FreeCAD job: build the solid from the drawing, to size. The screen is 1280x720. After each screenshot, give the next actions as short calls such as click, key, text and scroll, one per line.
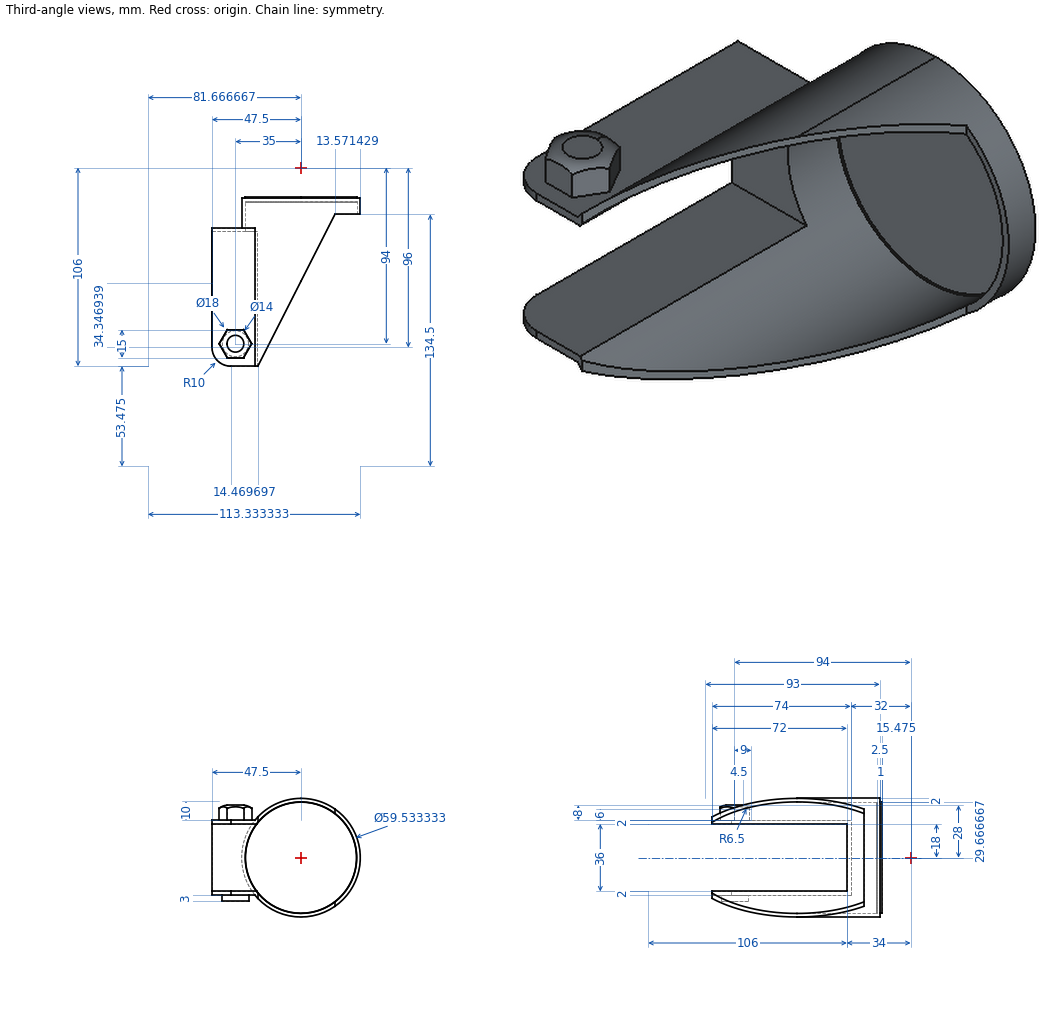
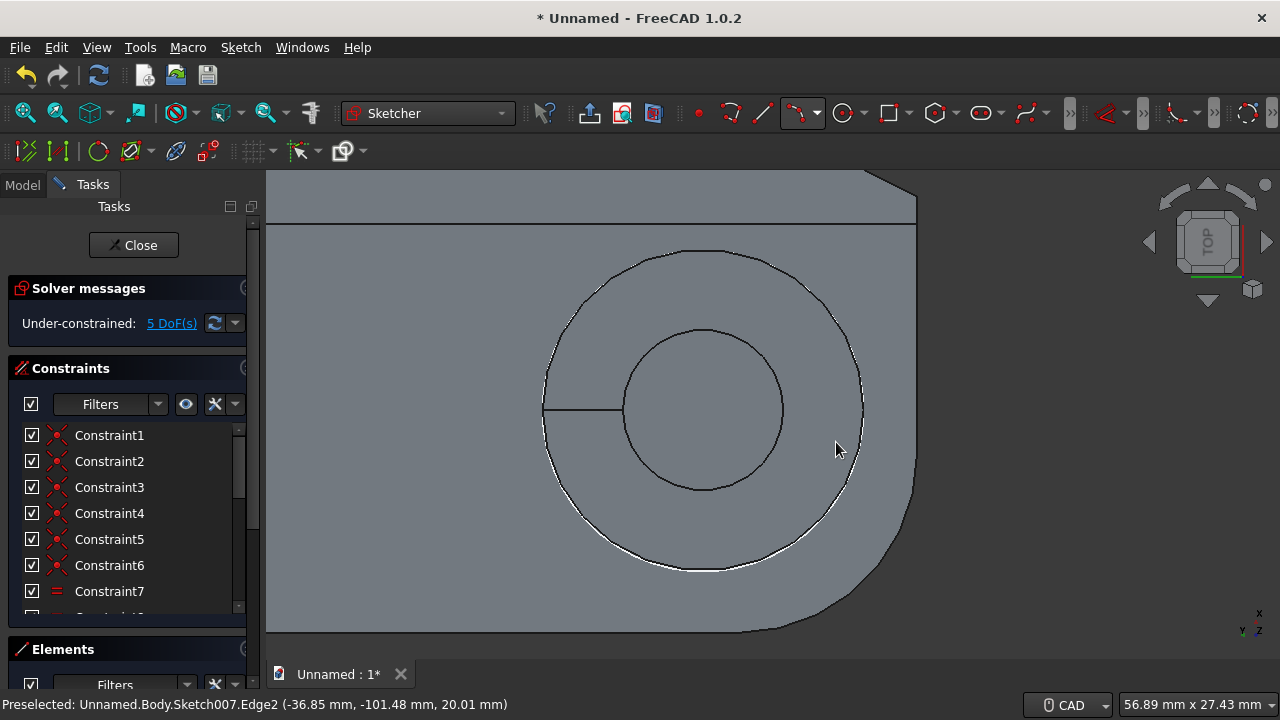
key(v)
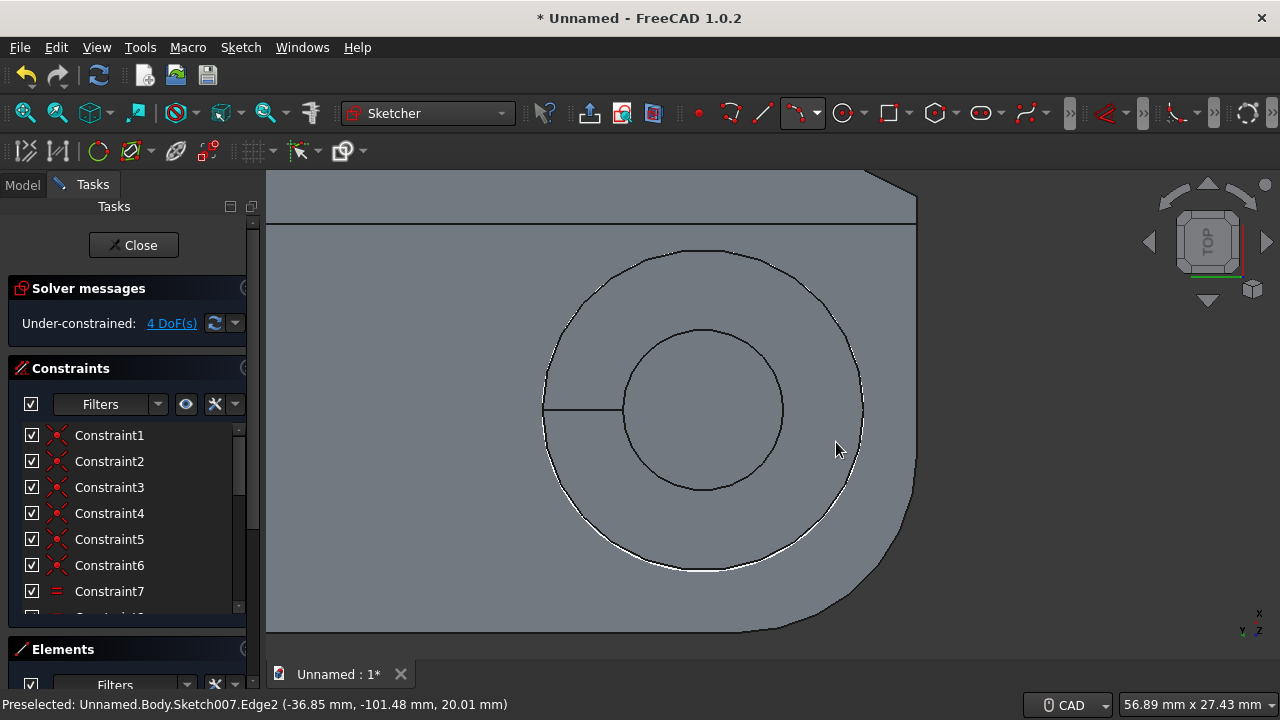
key(d)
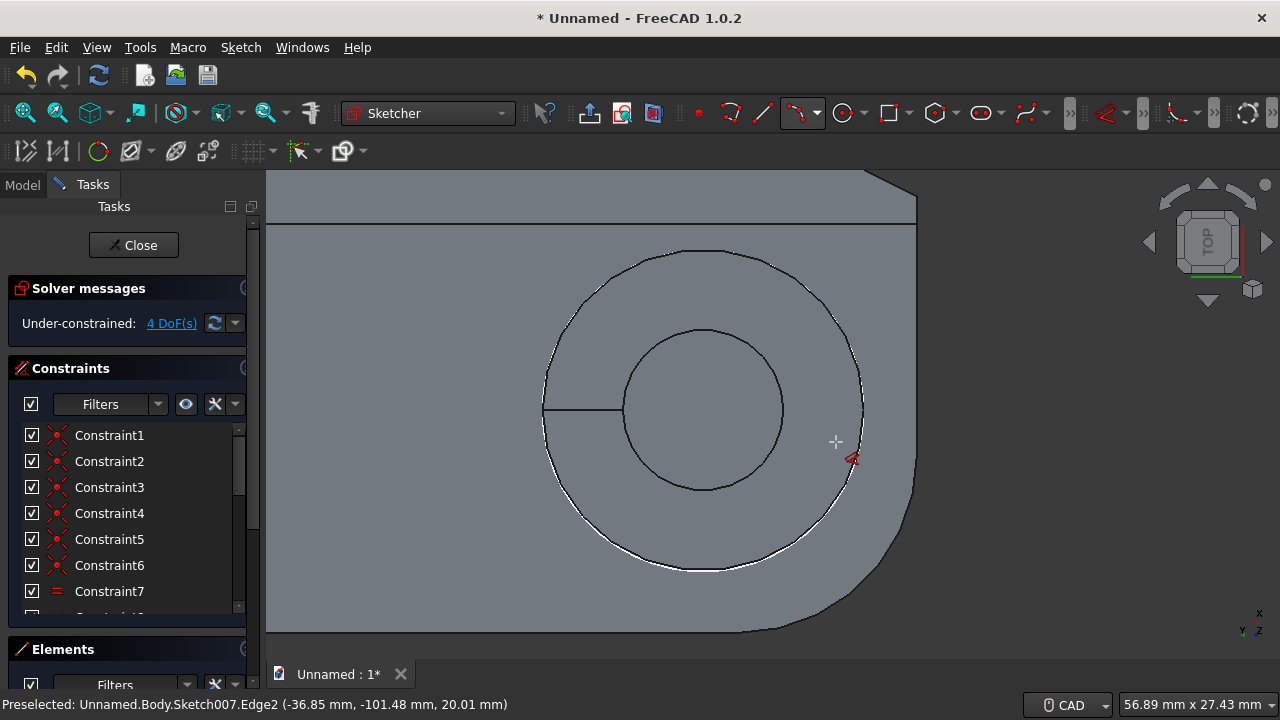
scroll(816, 297, up, 4)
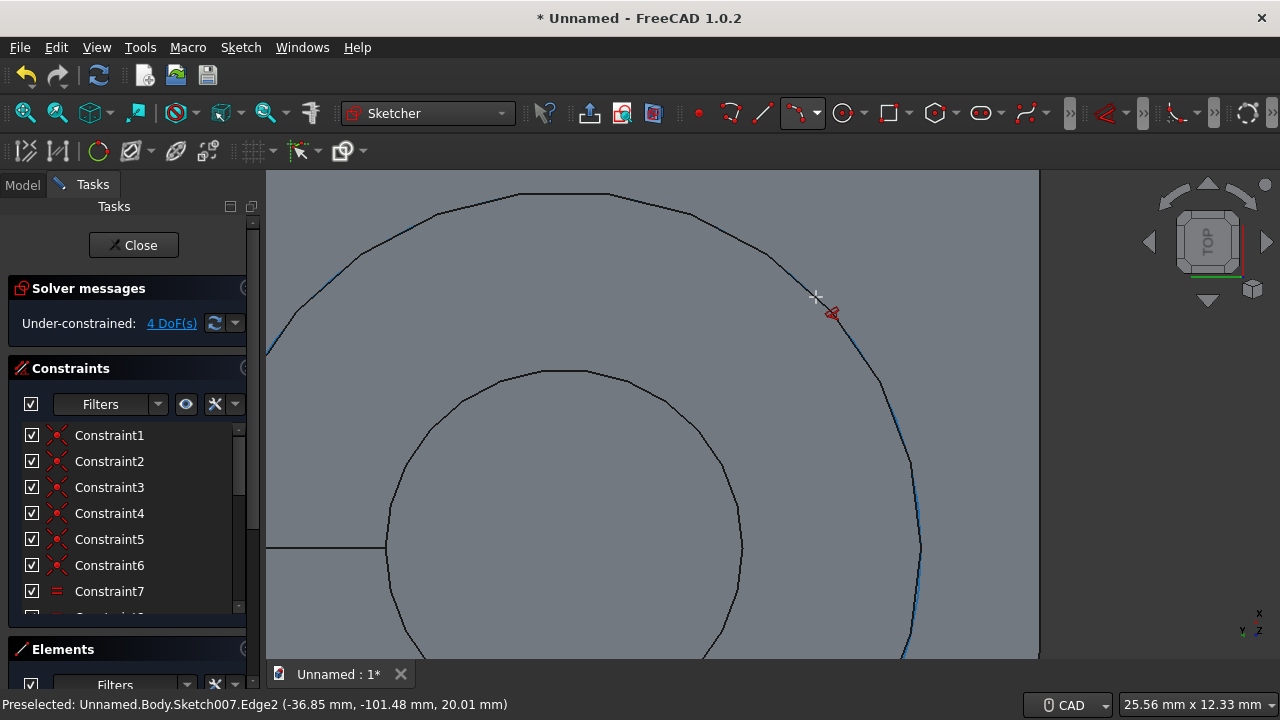
click(816, 297)
click(839, 274)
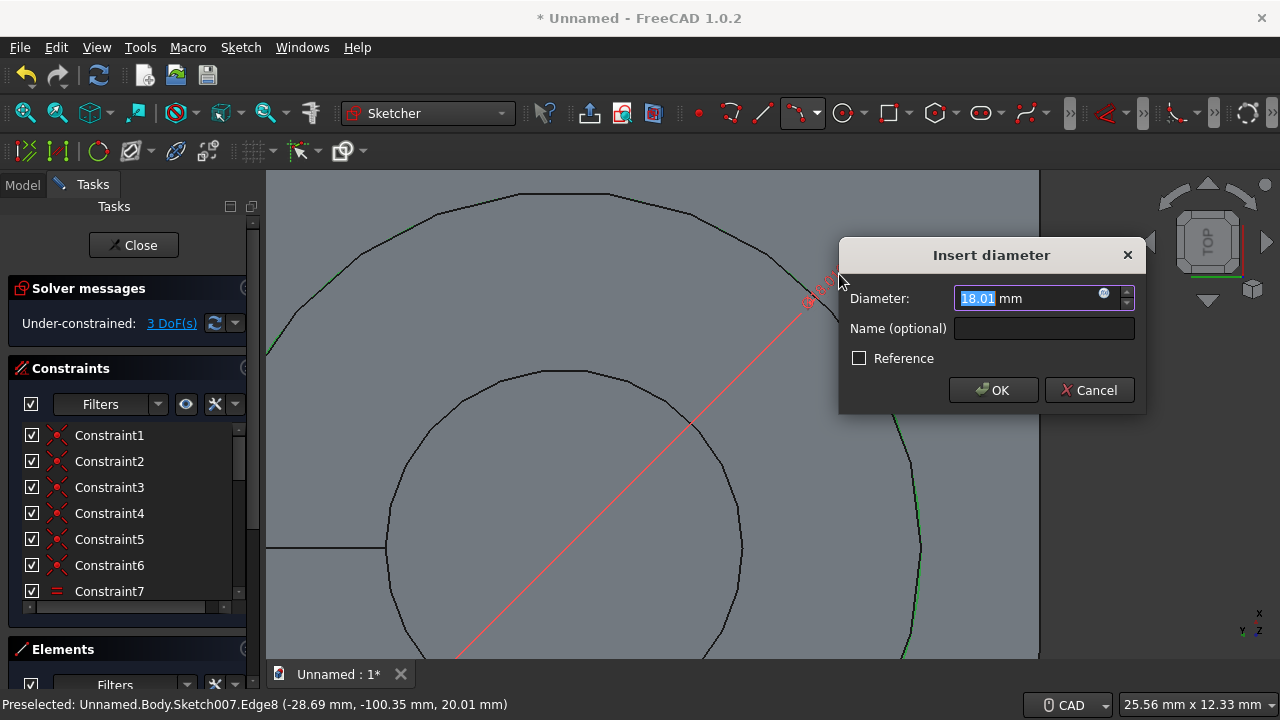
text(18)
key(Return)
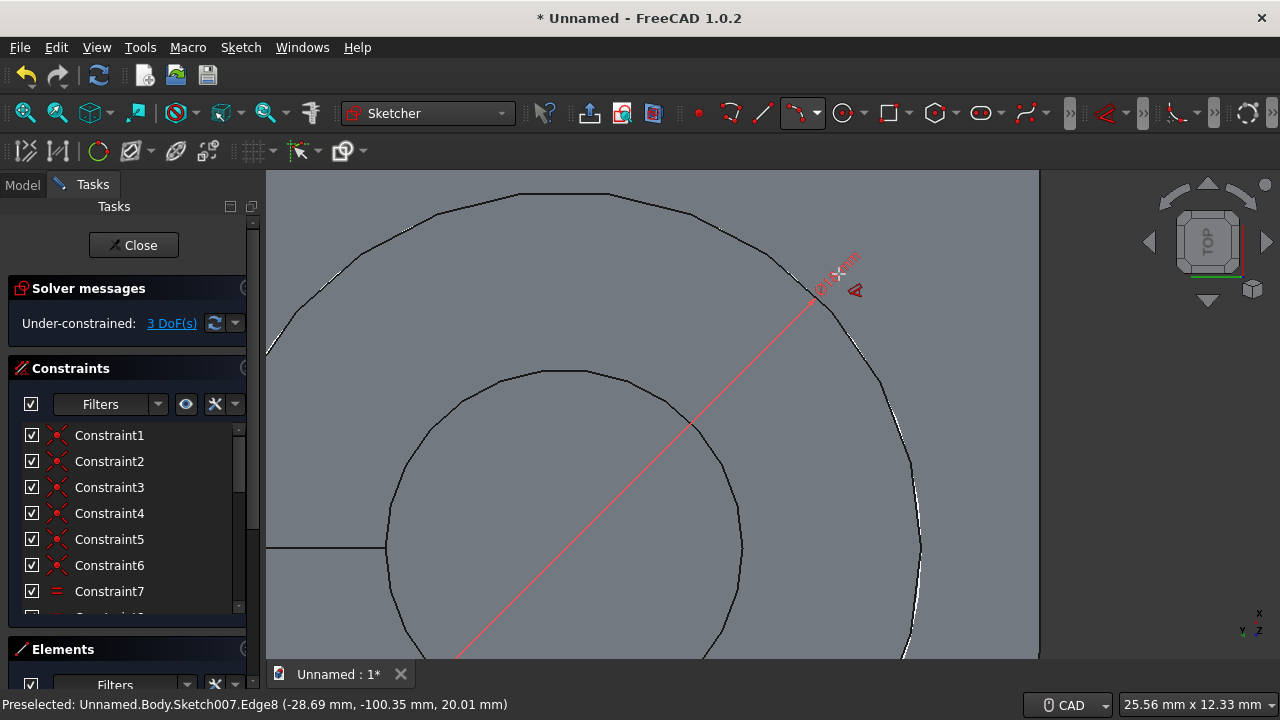
scroll(819, 305, down, 4)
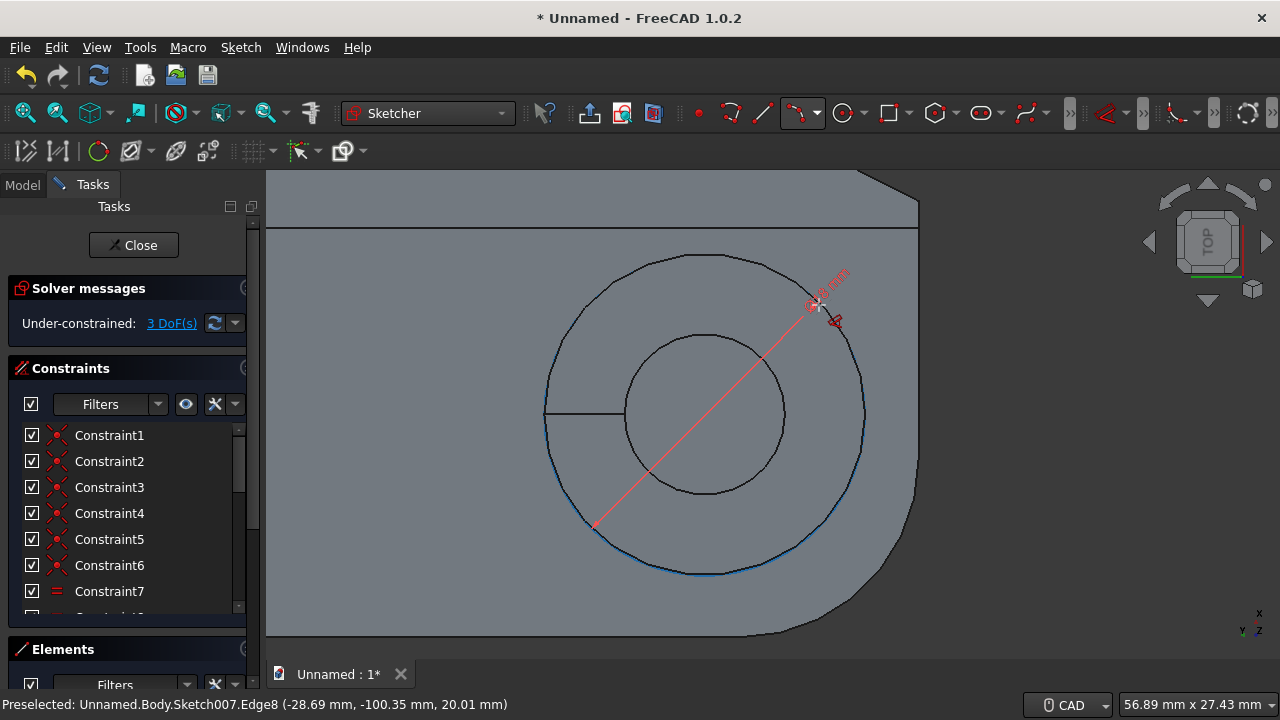
click(571, 338)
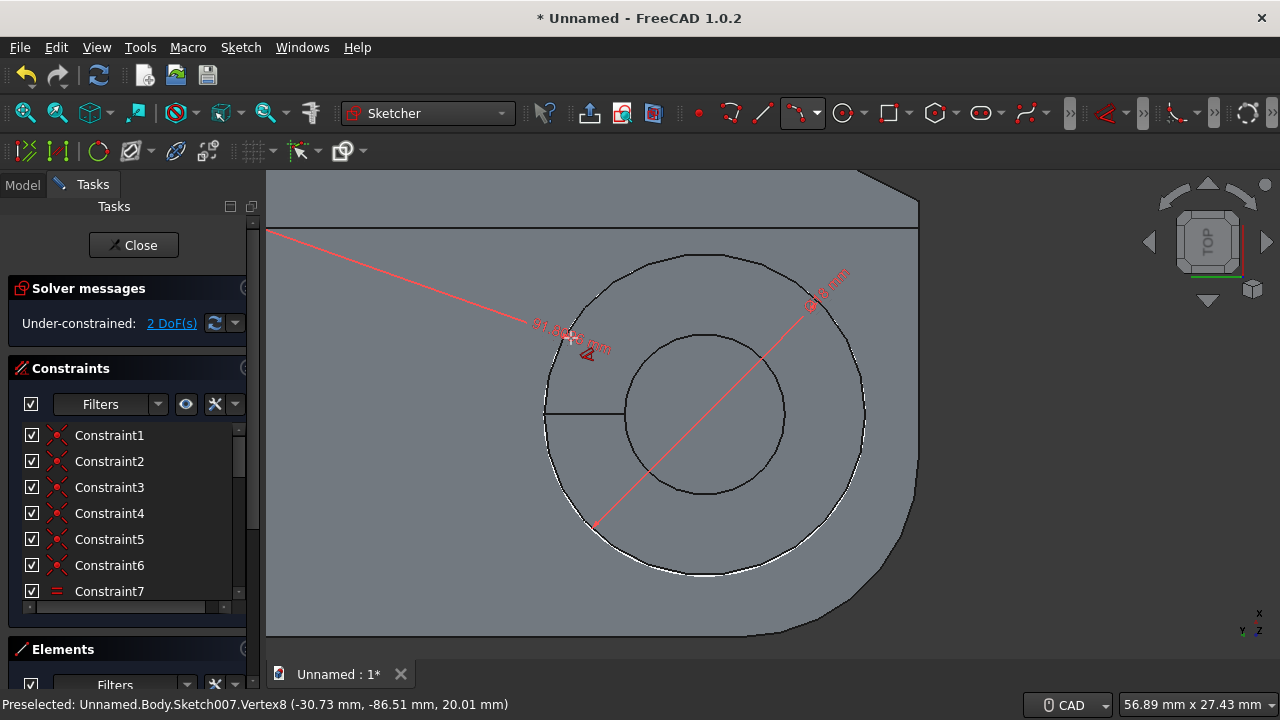
click(838, 492)
click(705, 526)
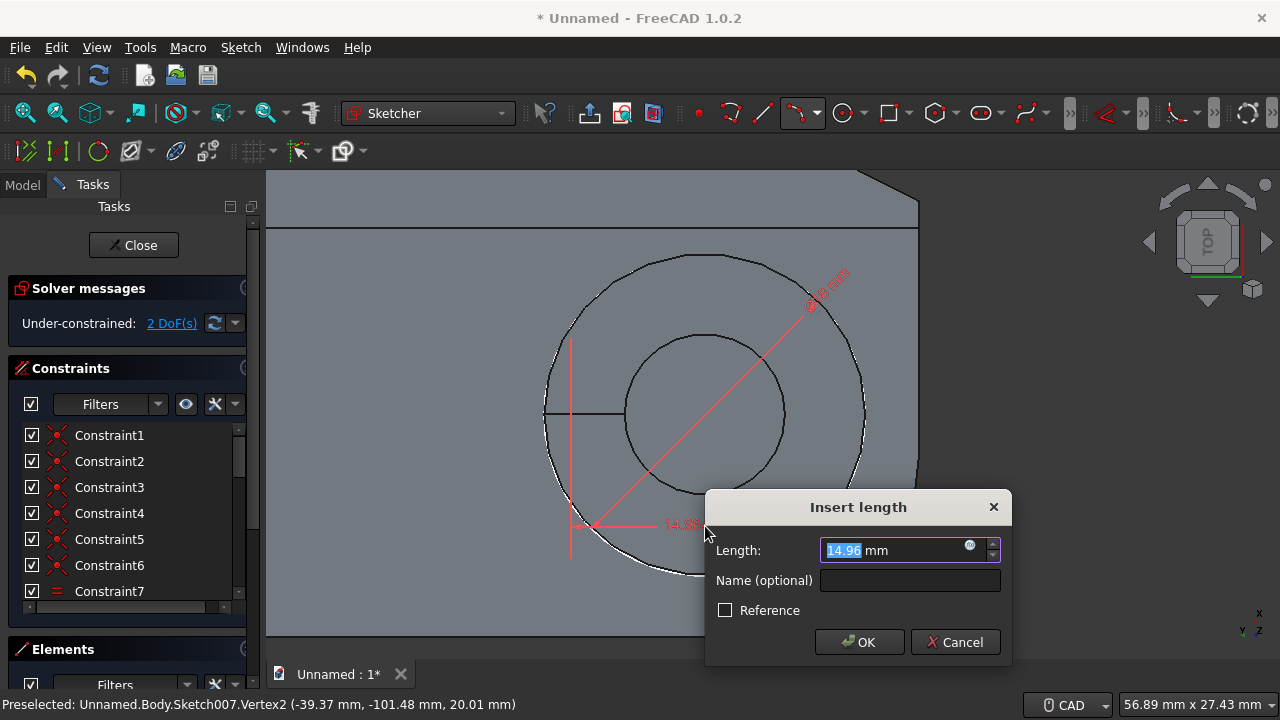
text(15)
key(Return)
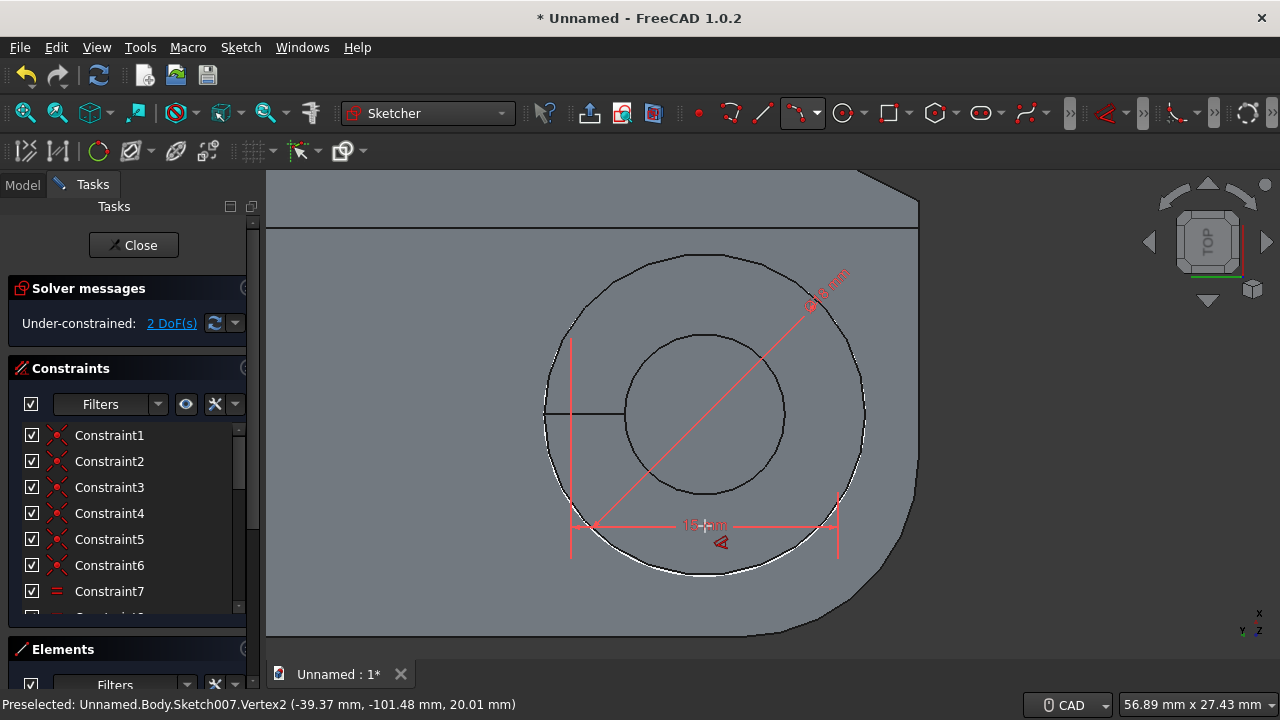
click(705, 416)
click(499, 450)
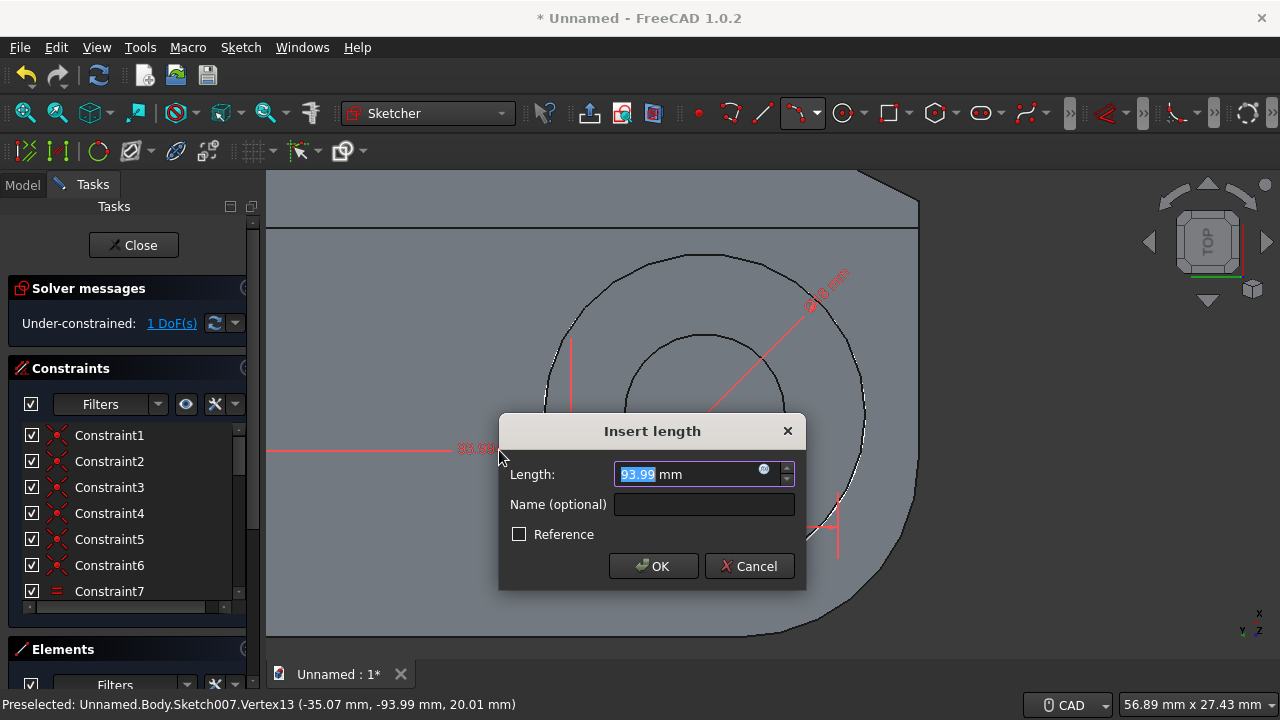
text(94)
key(Return)